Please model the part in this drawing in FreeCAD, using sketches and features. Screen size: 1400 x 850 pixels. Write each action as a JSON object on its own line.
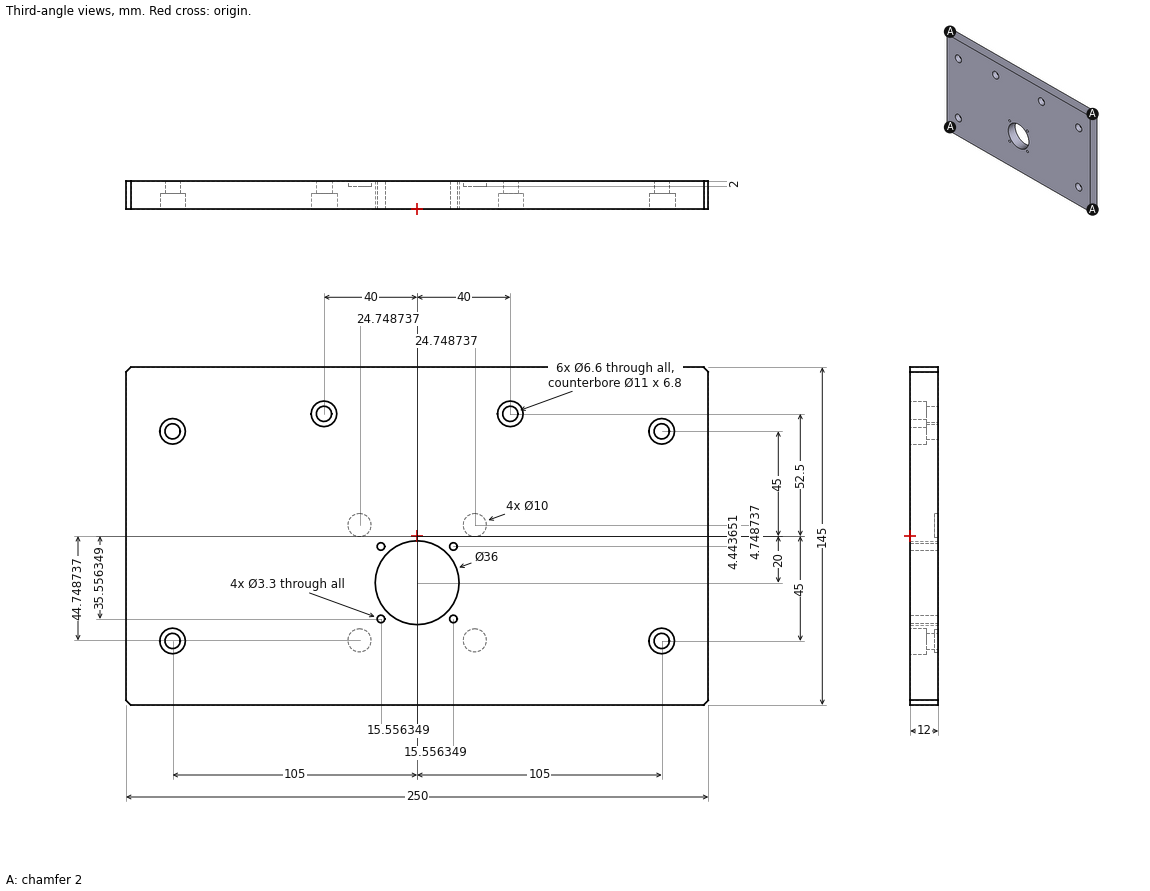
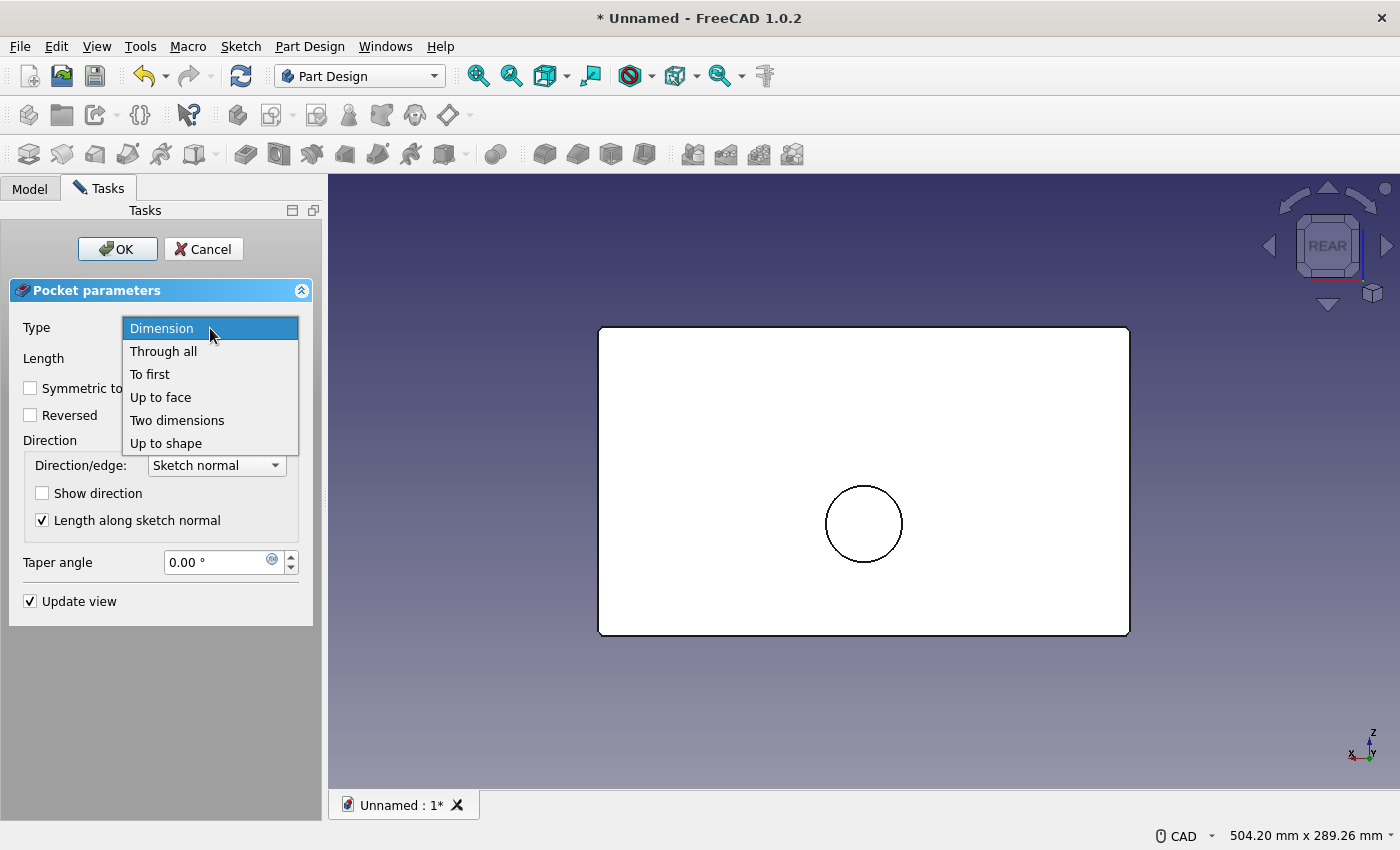
{"action": "left_click", "coordinate": [208, 352]}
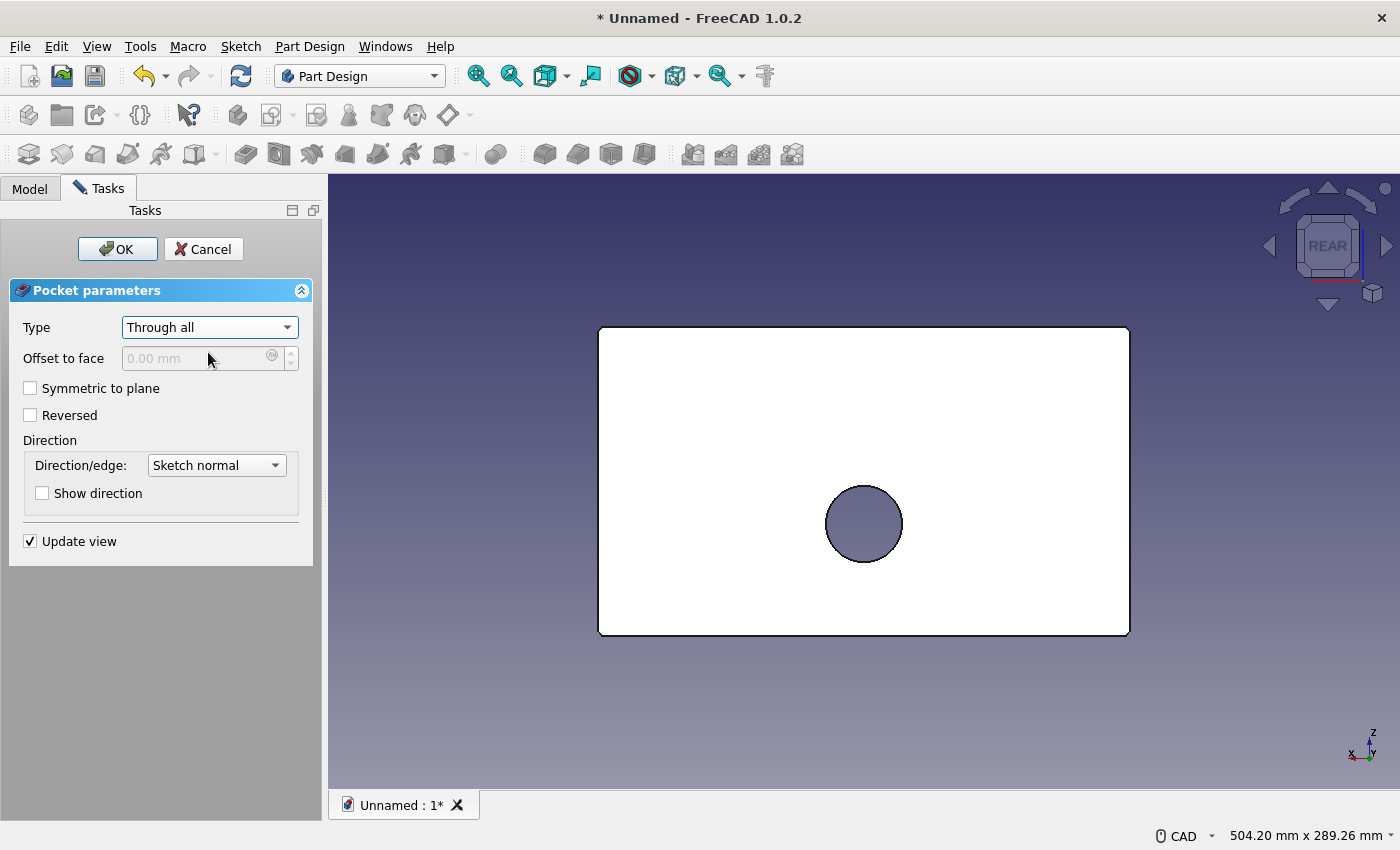
{"action": "left_click", "coordinate": [118, 249]}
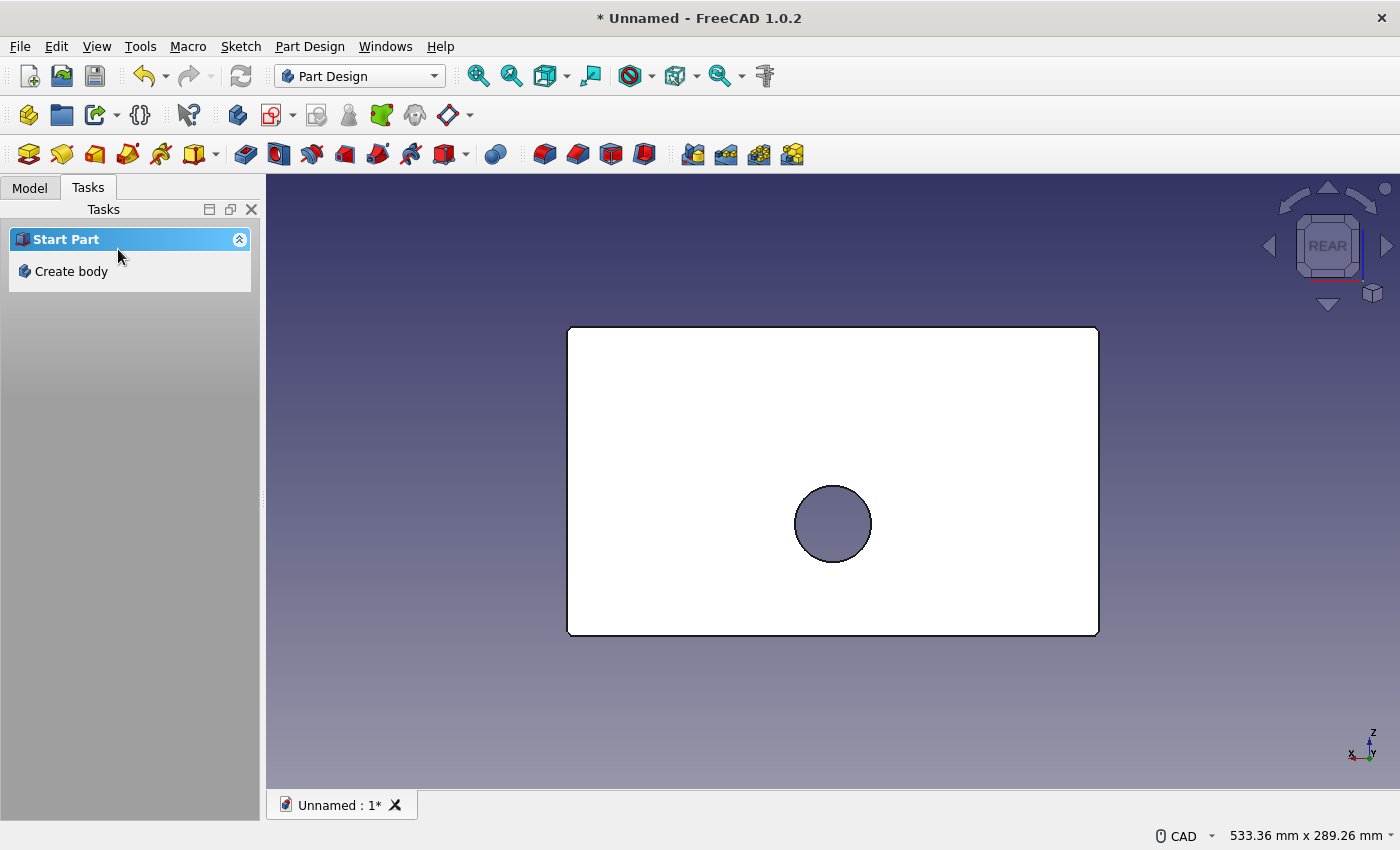
{"action": "left_click", "coordinate": [270, 116]}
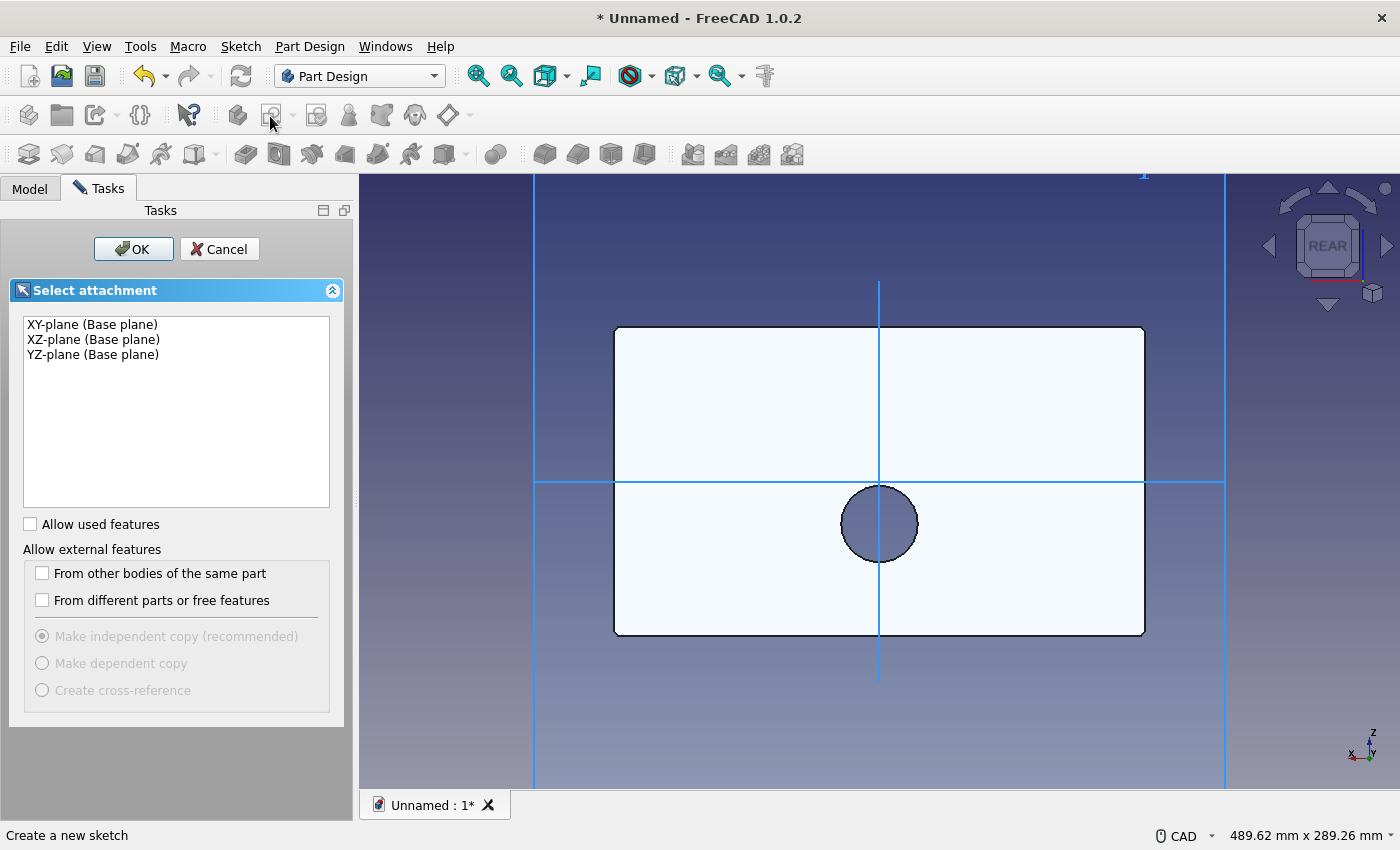
{"action": "left_click", "coordinate": [84, 340]}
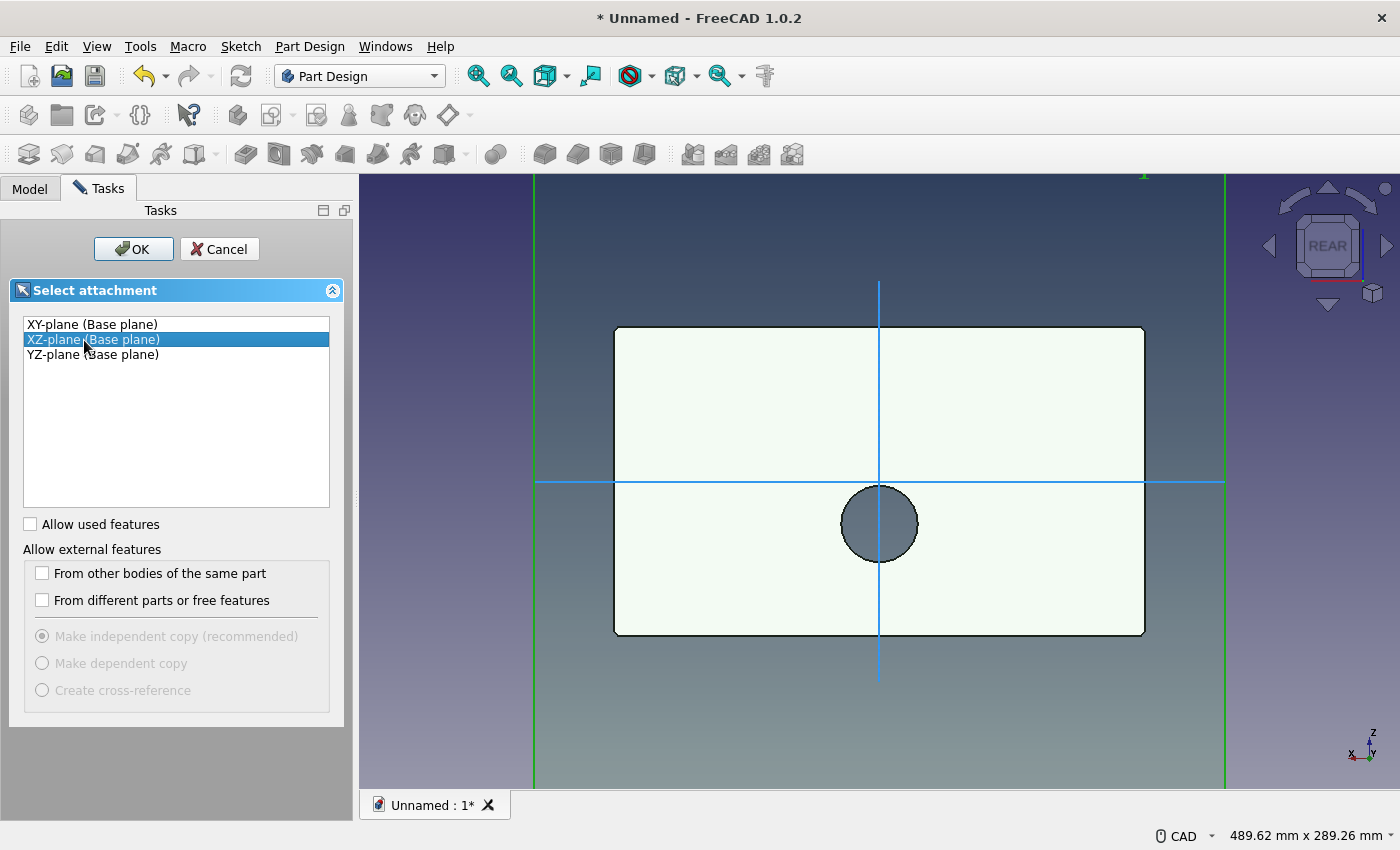
{"action": "left_click", "coordinate": [134, 249]}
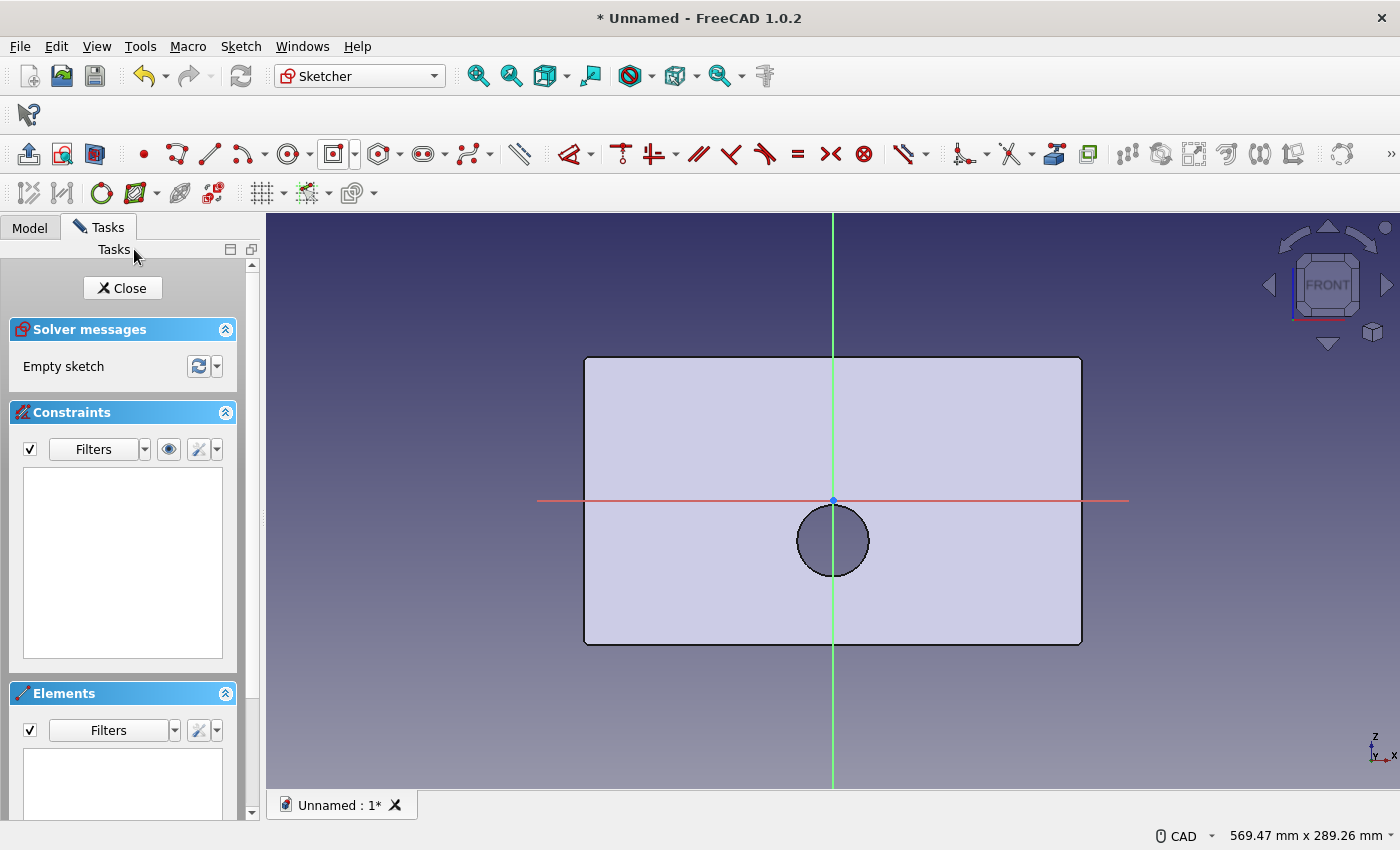
{"action": "scroll", "coordinate": [850, 547], "scroll_direction": "up", "scroll_amount": 8}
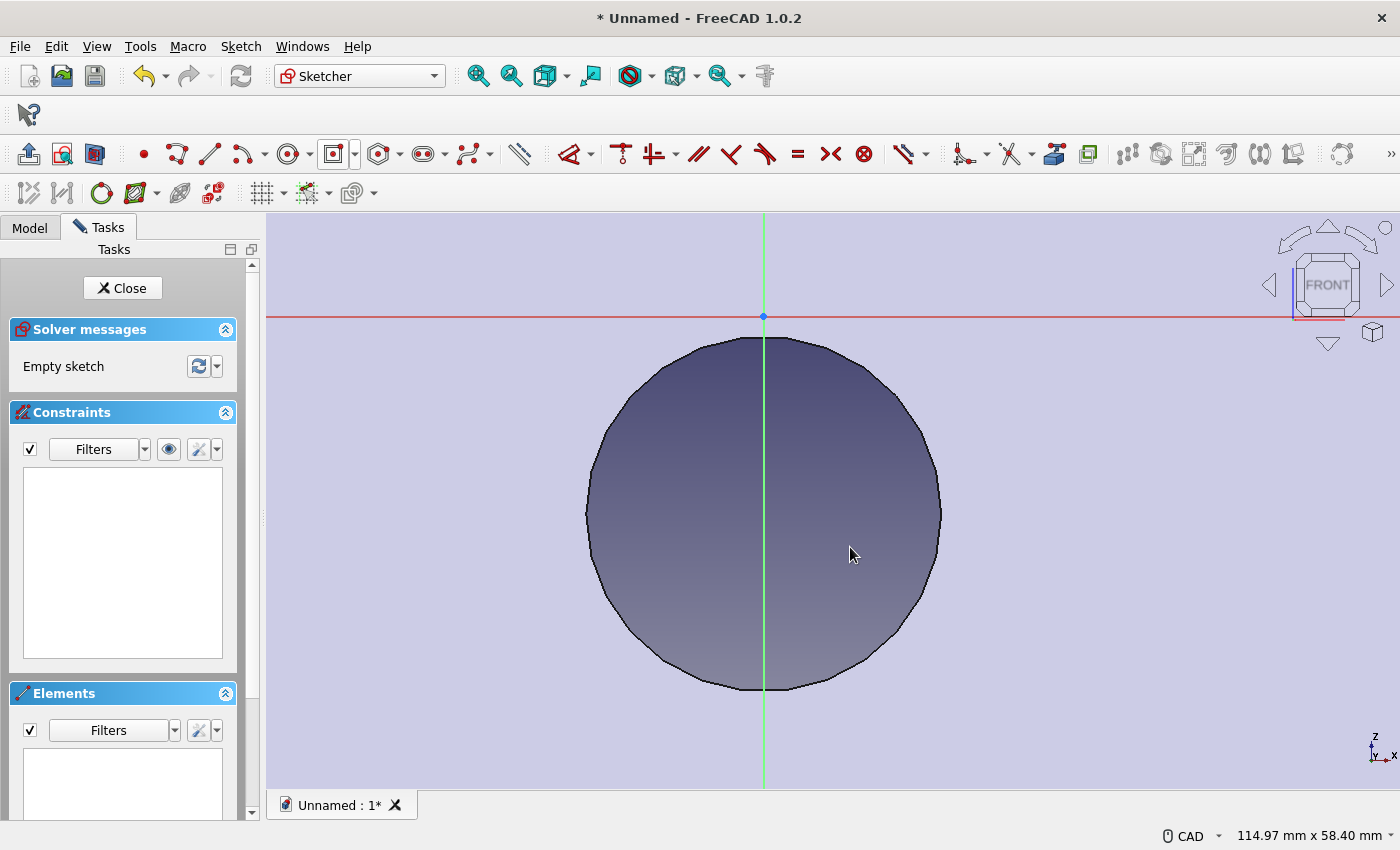
{"action": "left_click", "coordinate": [288, 154]}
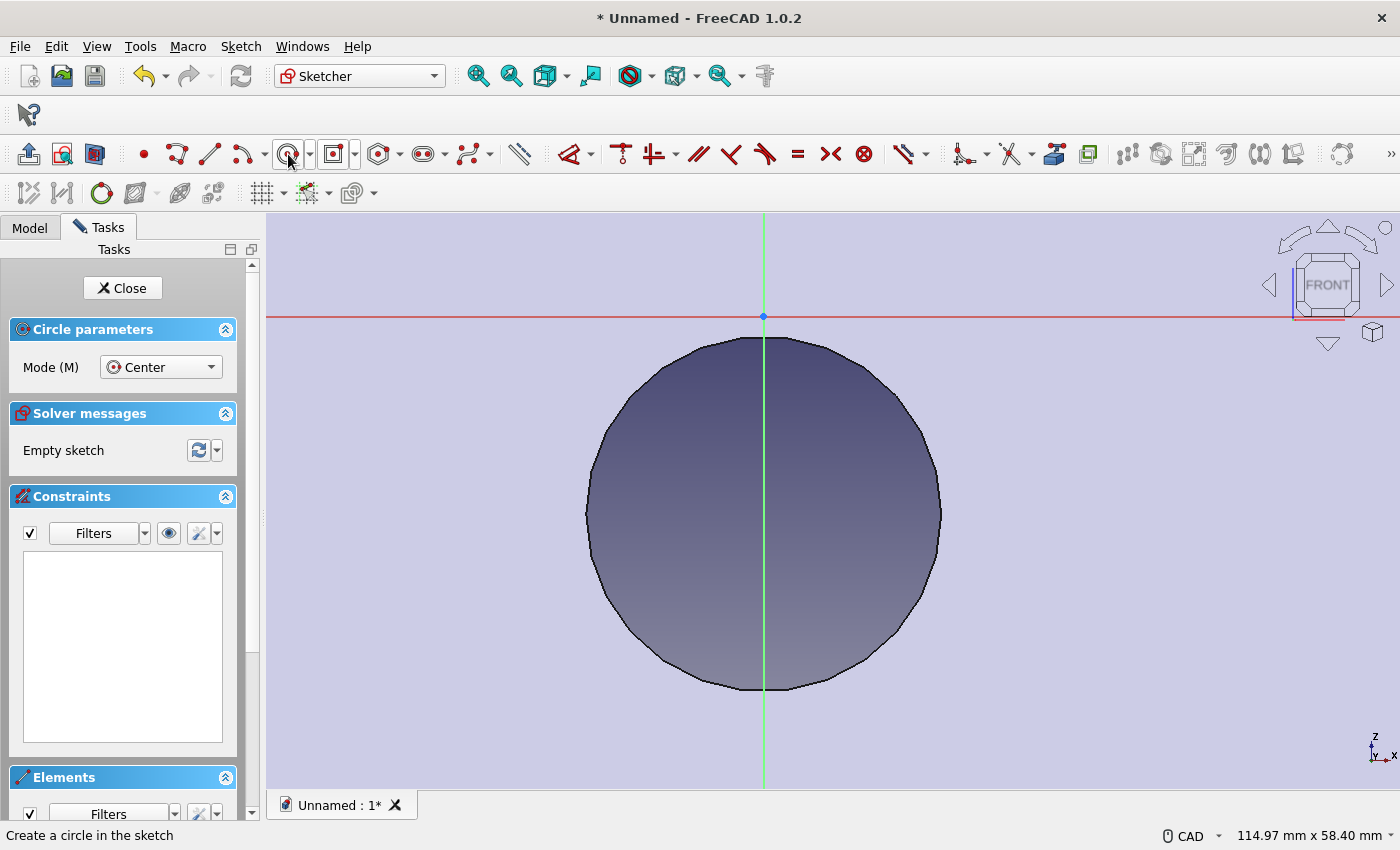
{"action": "scroll", "coordinate": [610, 668], "scroll_direction": "up", "scroll_amount": 2}